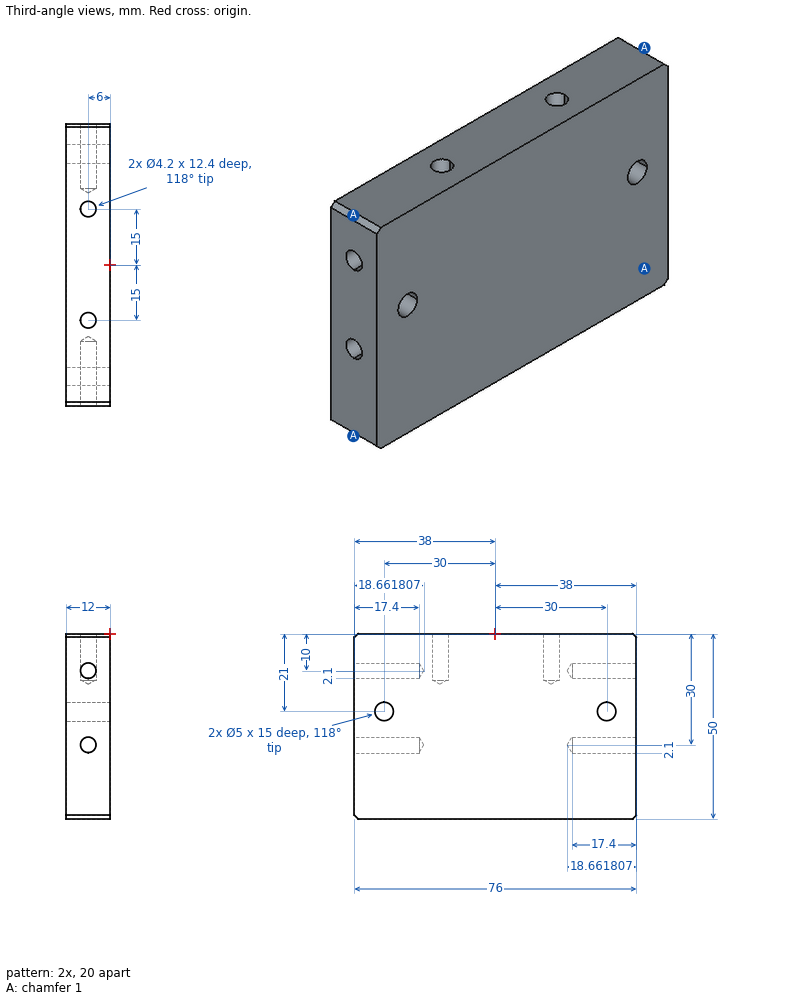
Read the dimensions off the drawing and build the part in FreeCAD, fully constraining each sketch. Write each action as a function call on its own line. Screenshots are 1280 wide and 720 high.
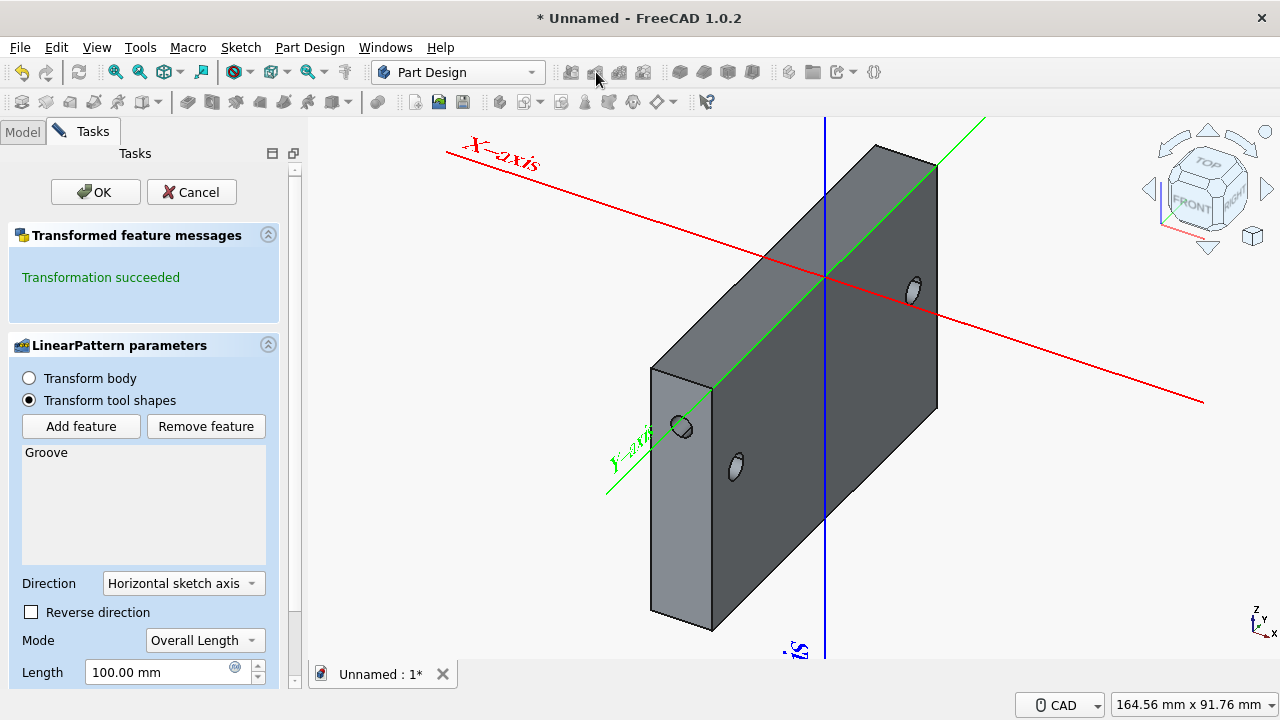
click(184, 584)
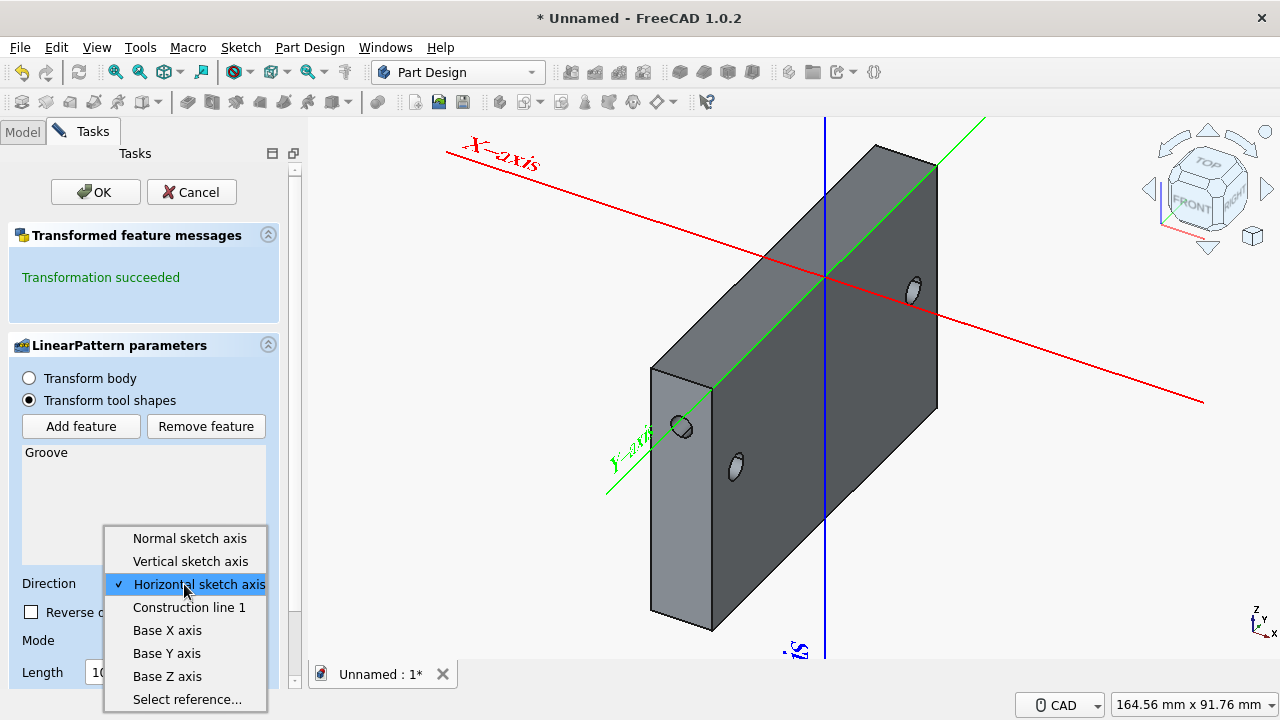
click(184, 676)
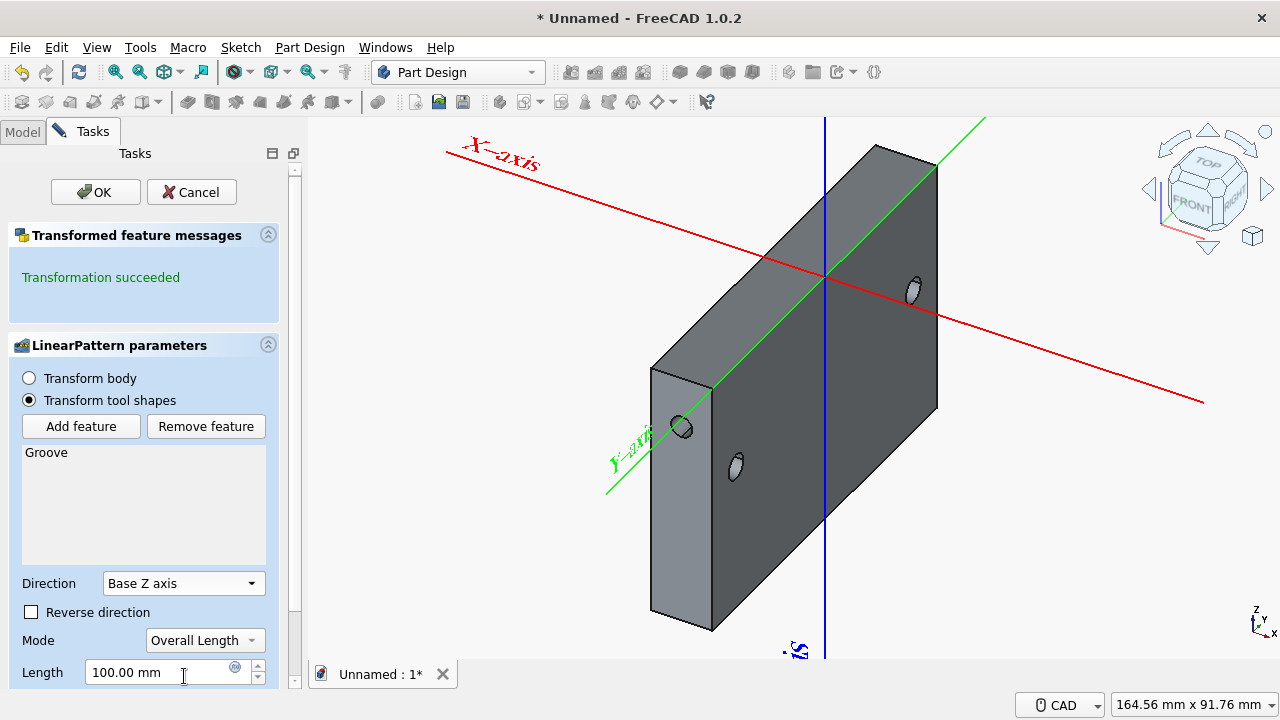
click(206, 640)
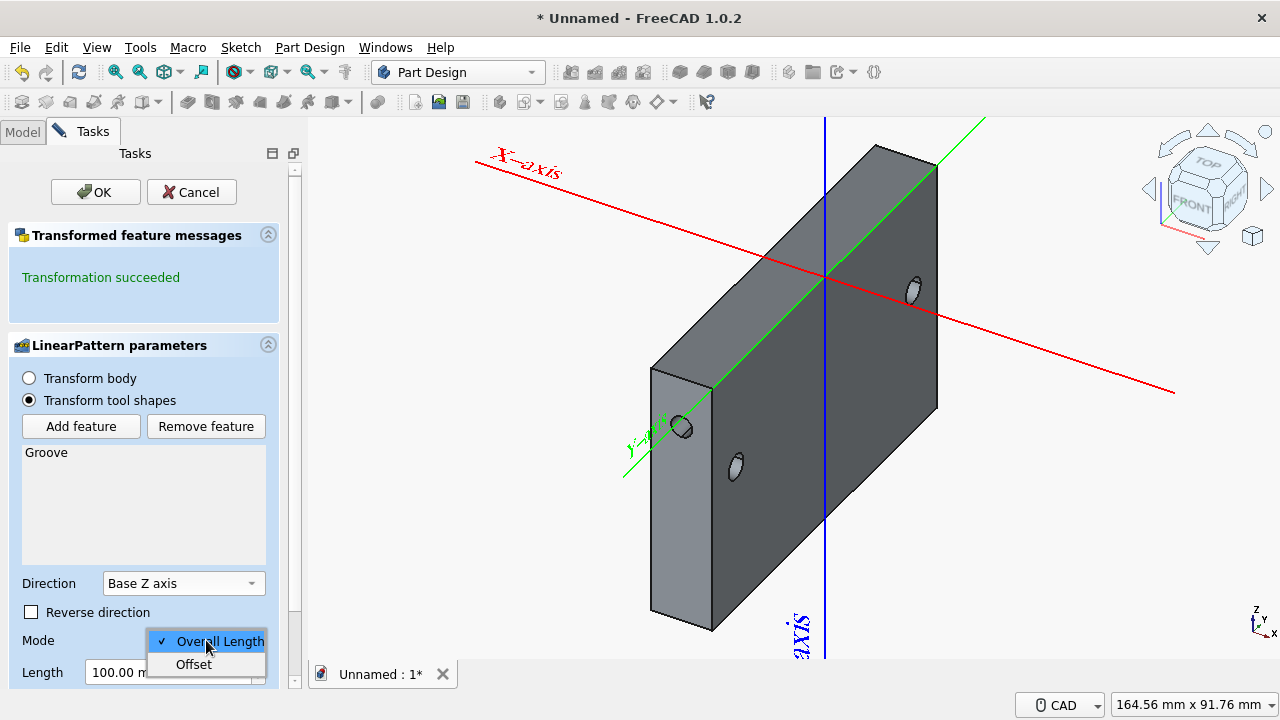
click(206, 664)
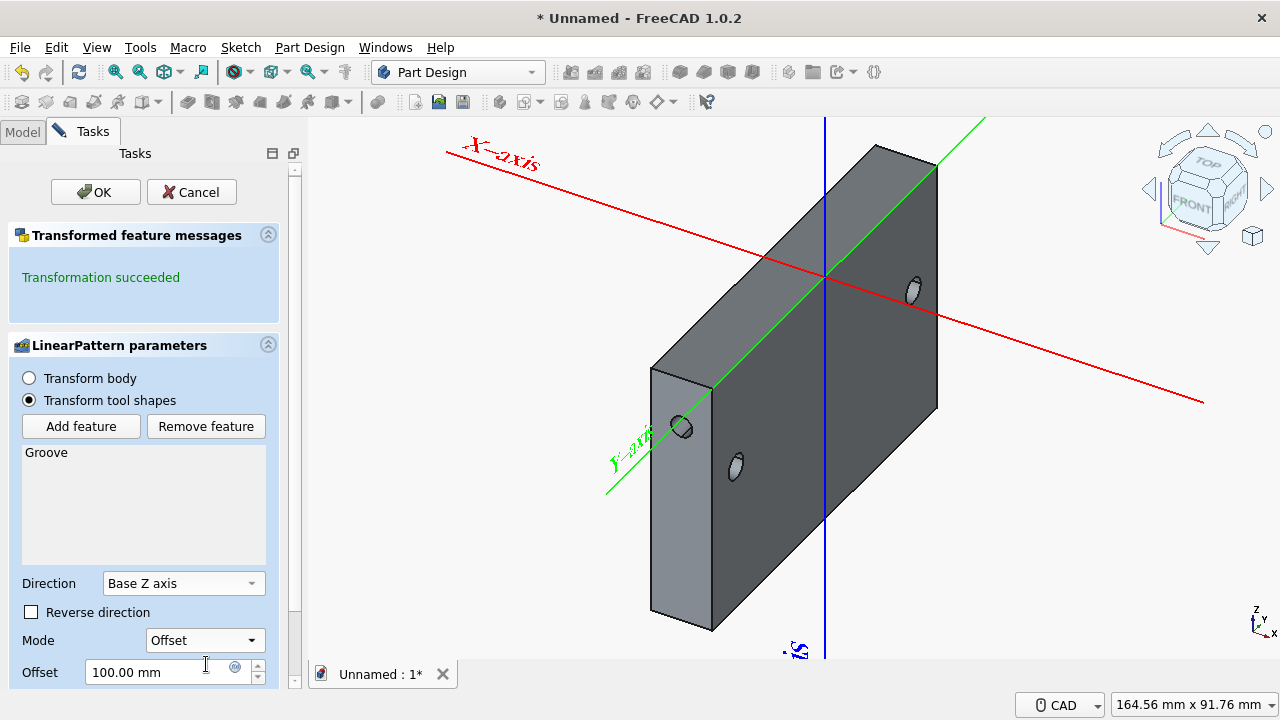
triple_click(168, 672)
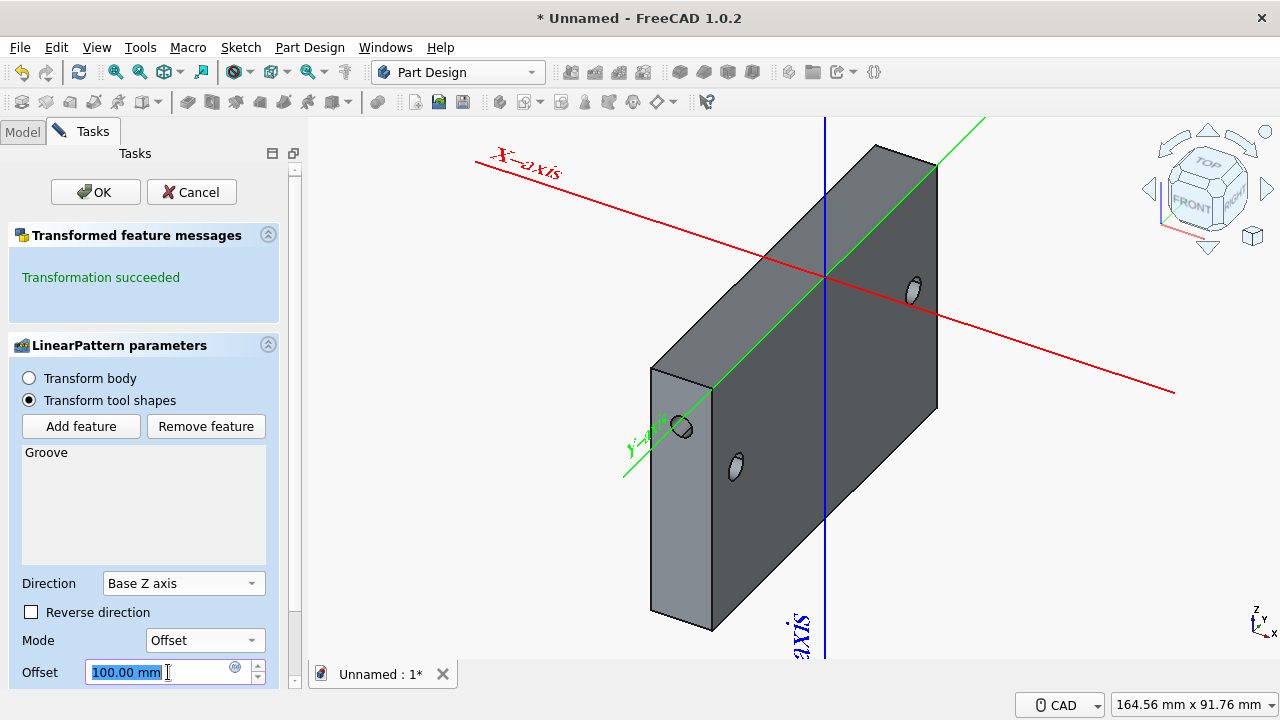
text(20)
key(Tab)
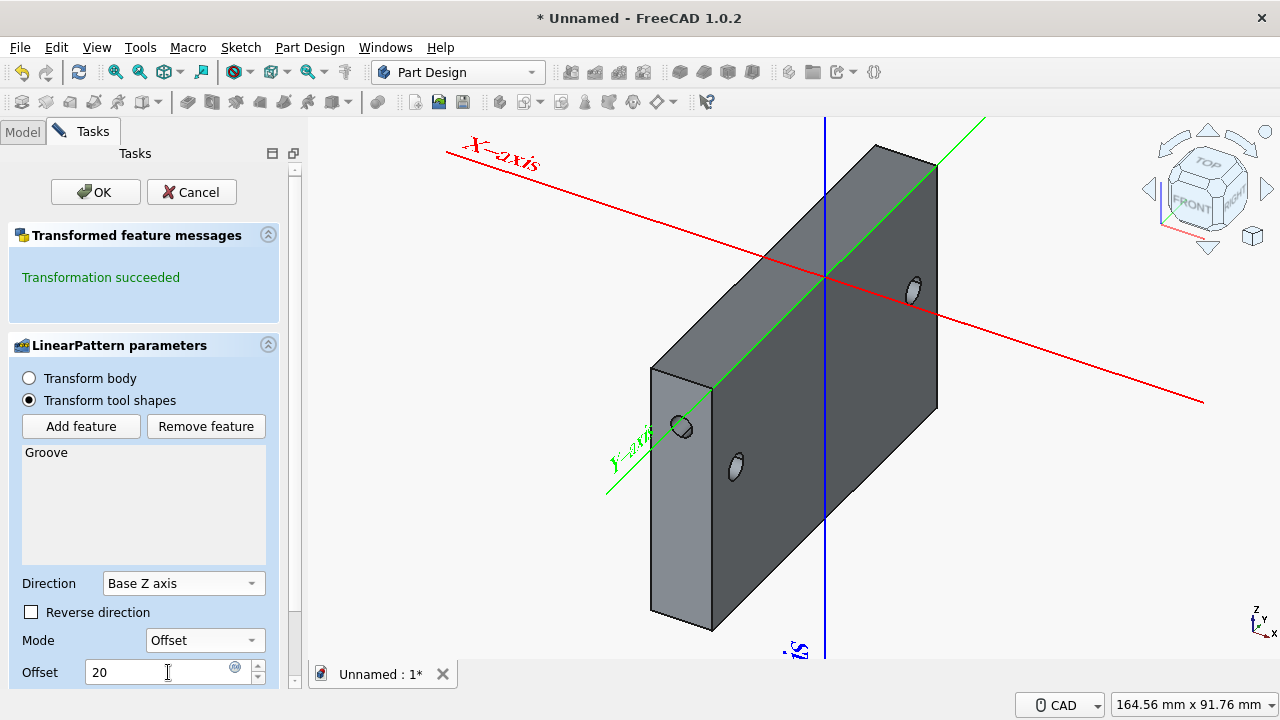
scroll(295, 426, down, 2)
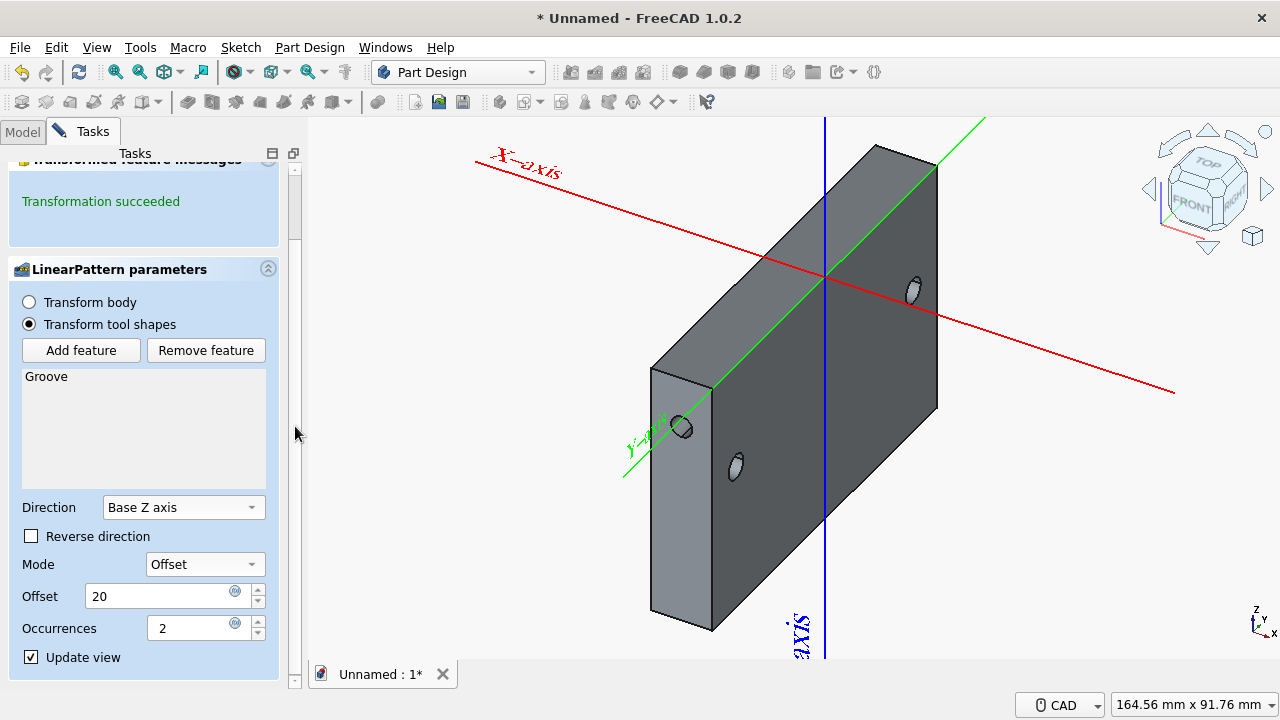
triple_click(198, 628)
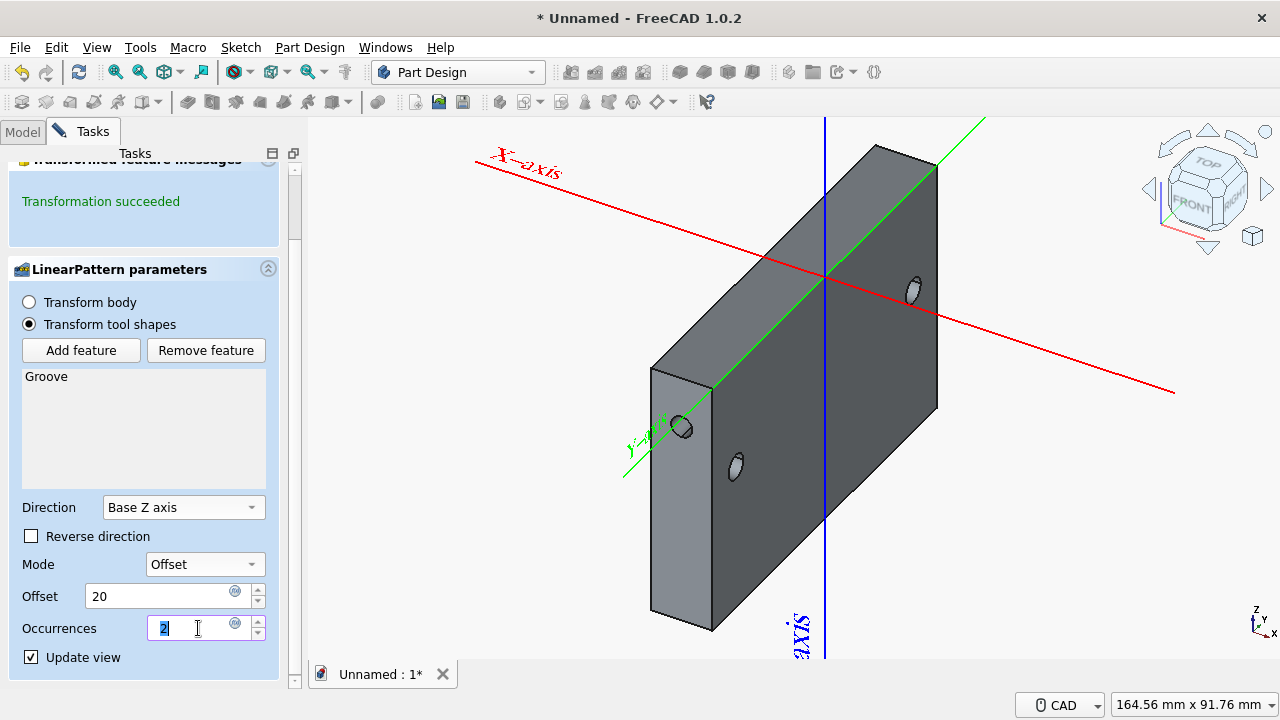
text(2)
key(Tab)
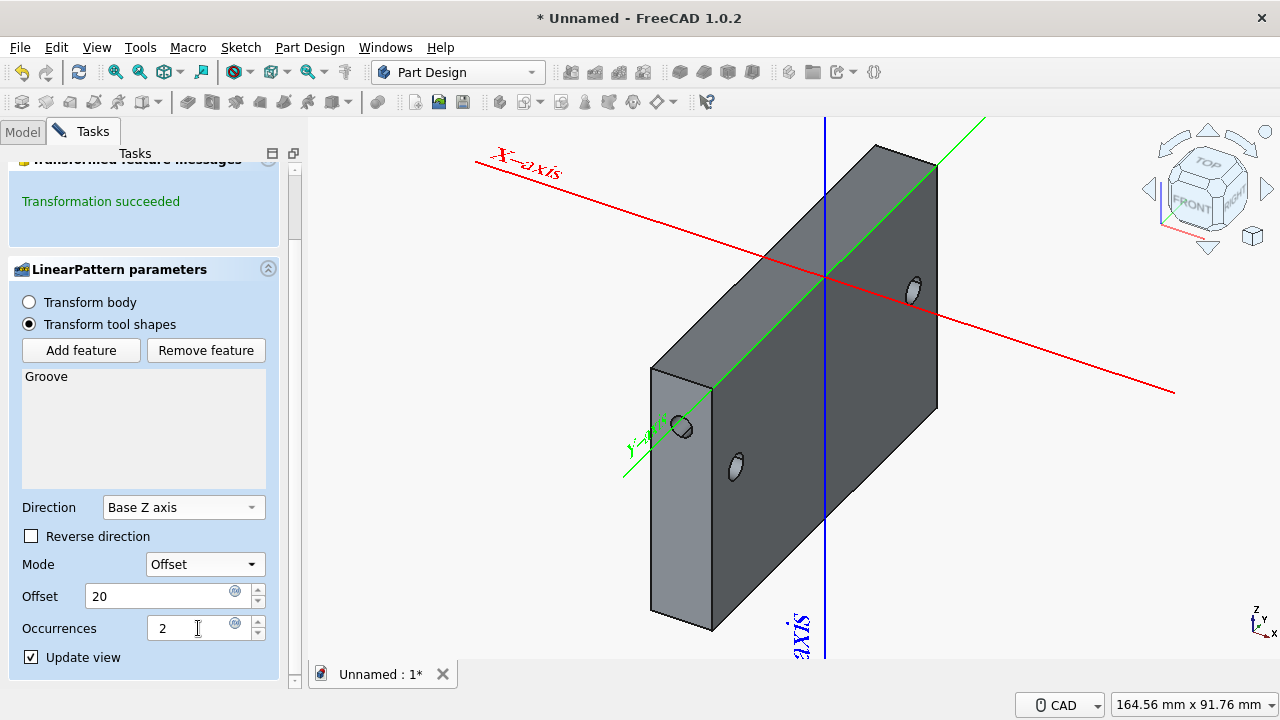
click(30, 536)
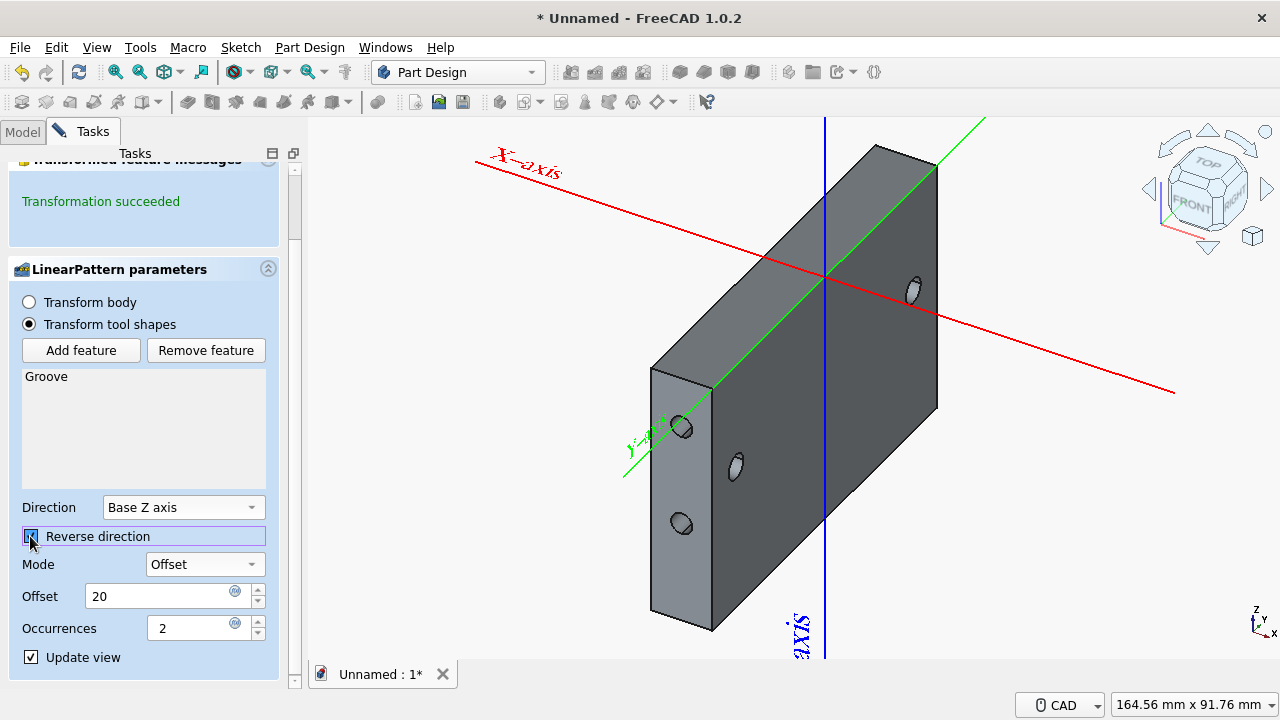
scroll(295, 426, up, 3)